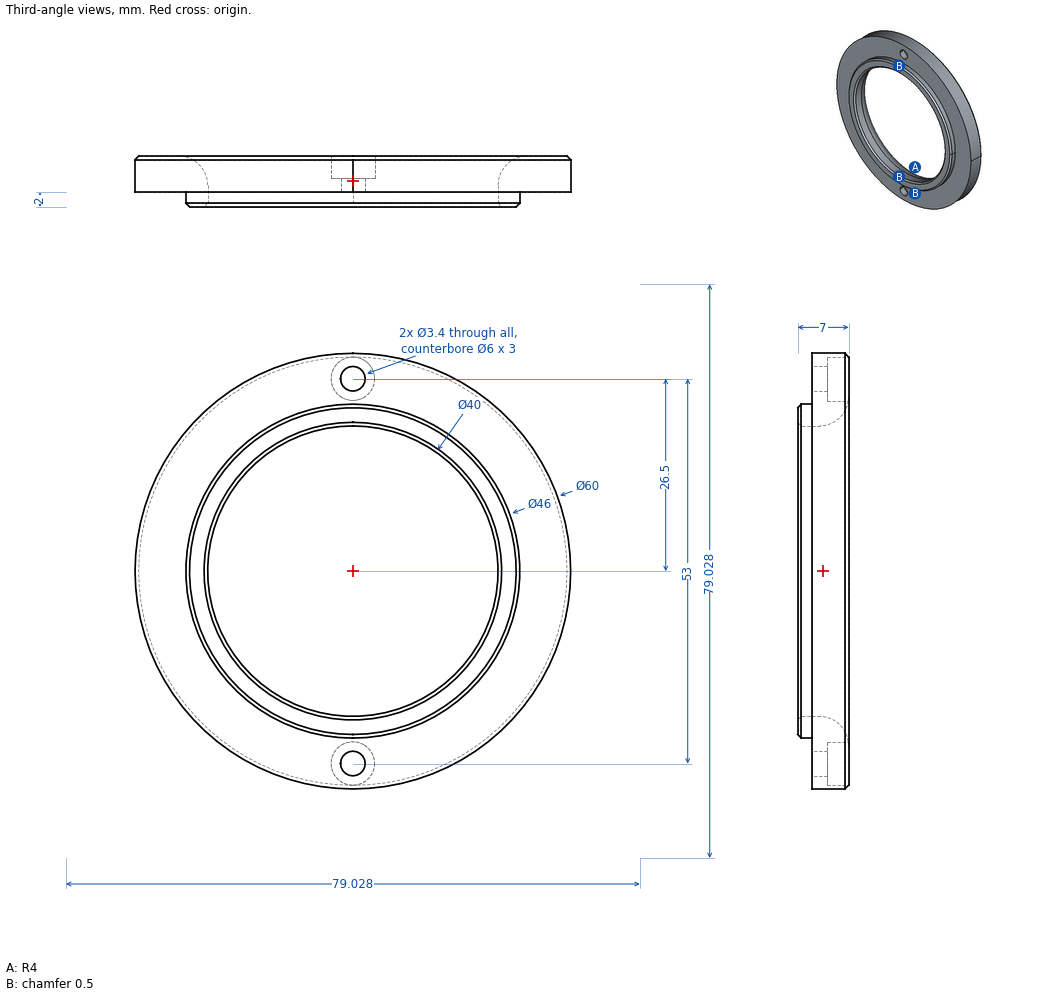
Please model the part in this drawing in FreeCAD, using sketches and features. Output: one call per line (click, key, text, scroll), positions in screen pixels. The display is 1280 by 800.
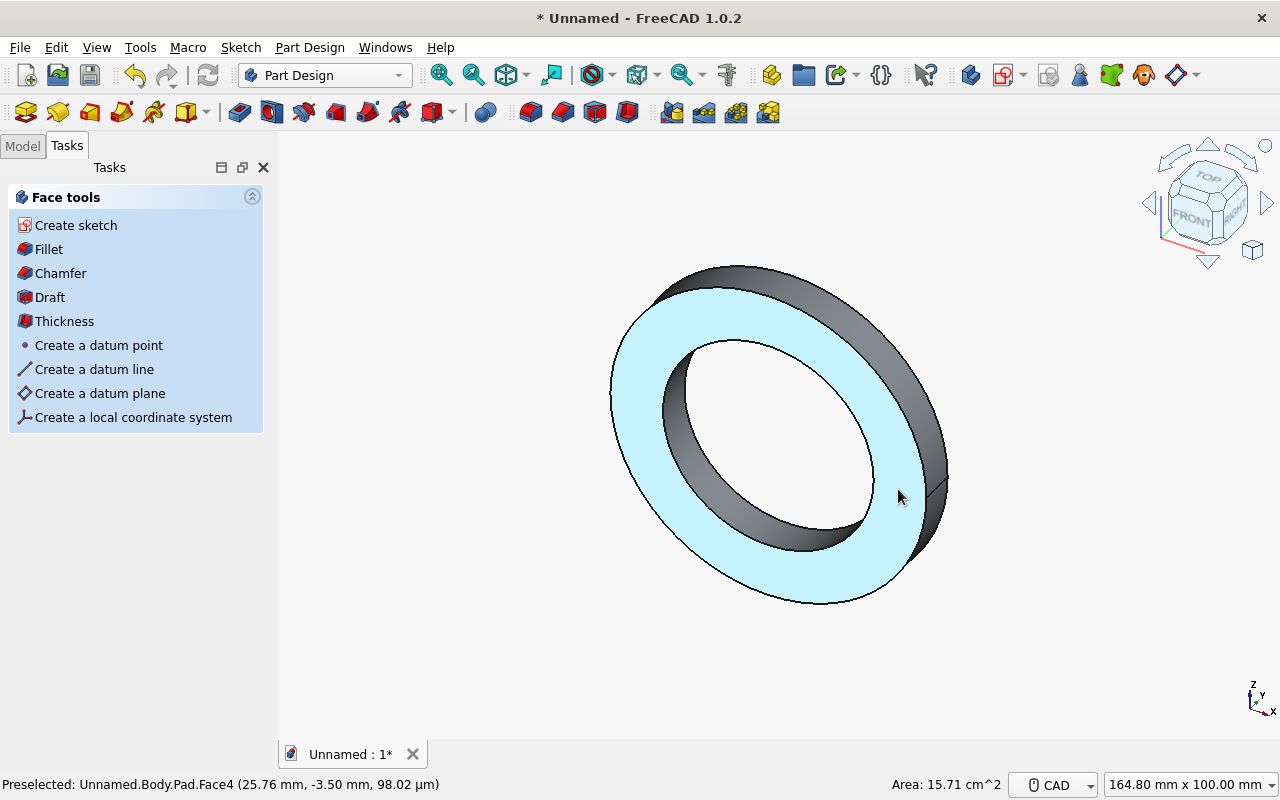
click(1004, 76)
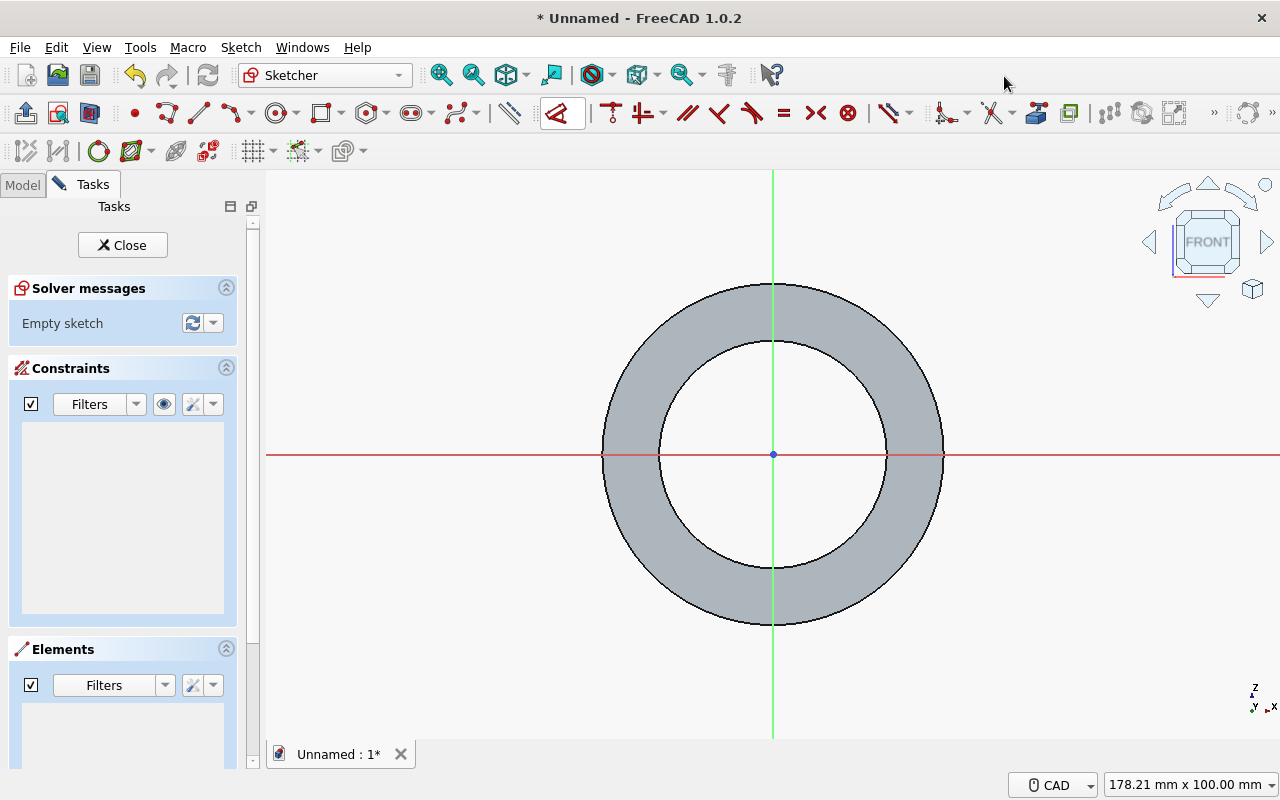
click(344, 114)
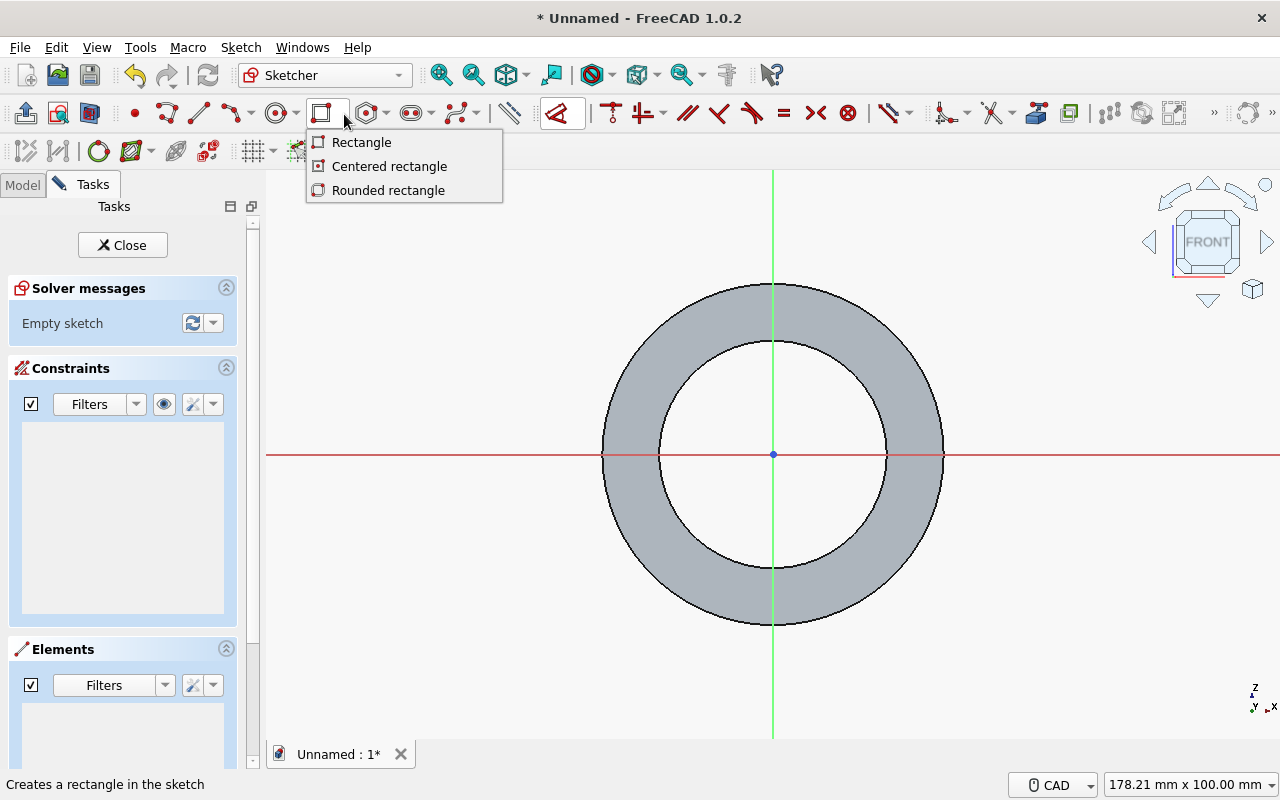
click(404, 166)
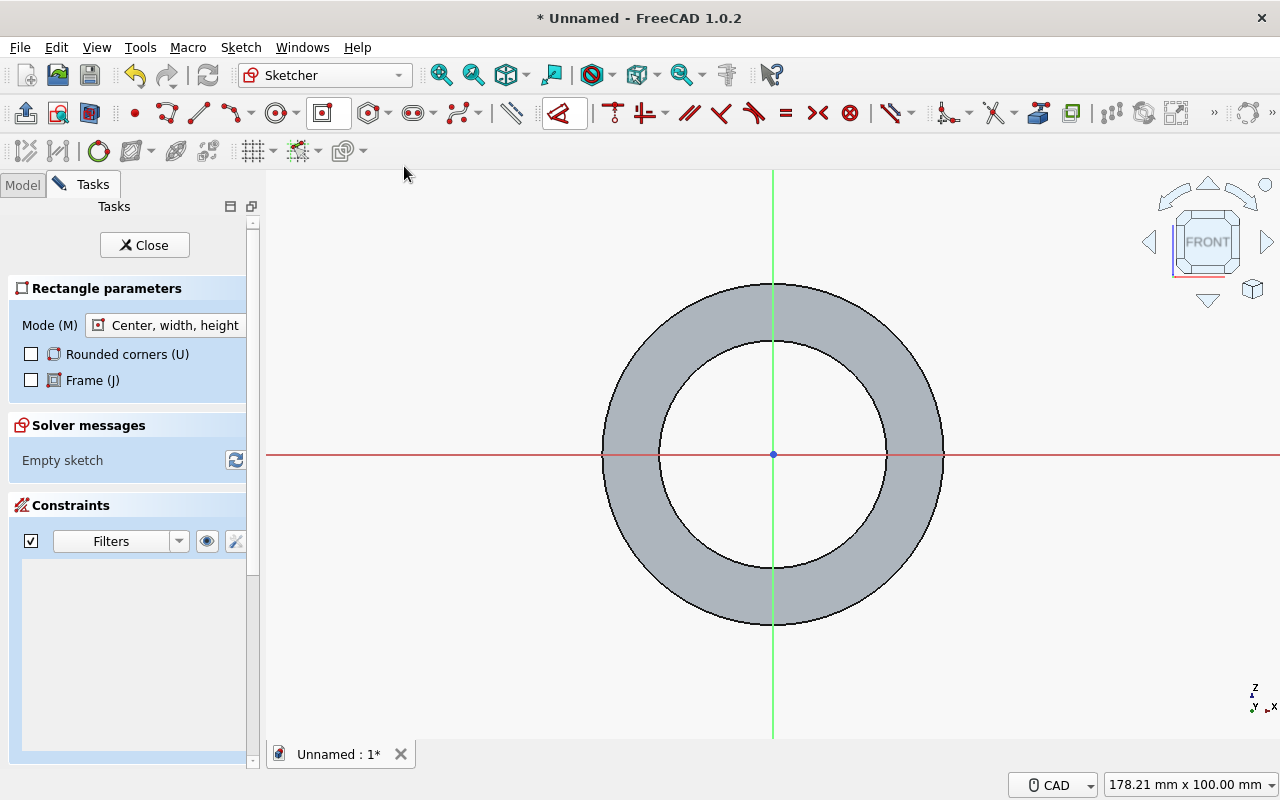
click(773, 454)
click(998, 230)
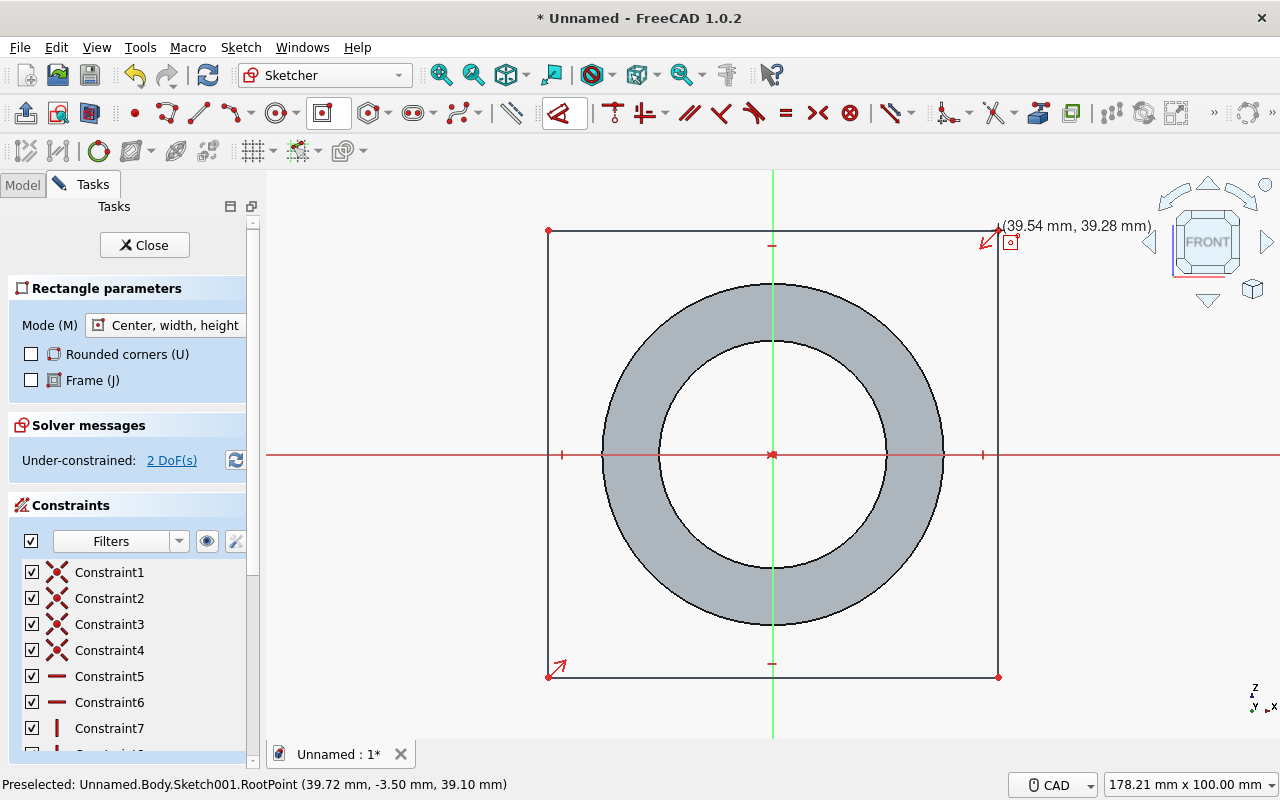
click(276, 114)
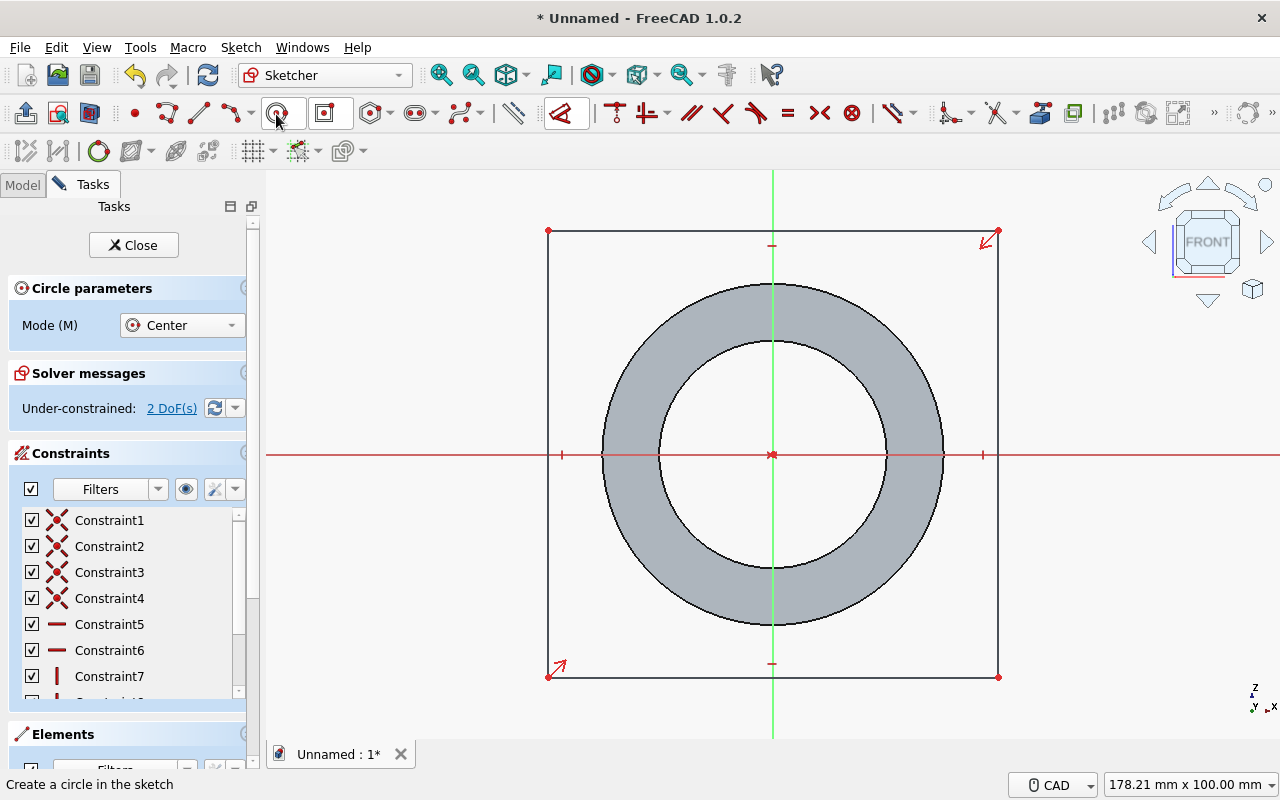
click(773, 454)
click(866, 362)
key(Escape)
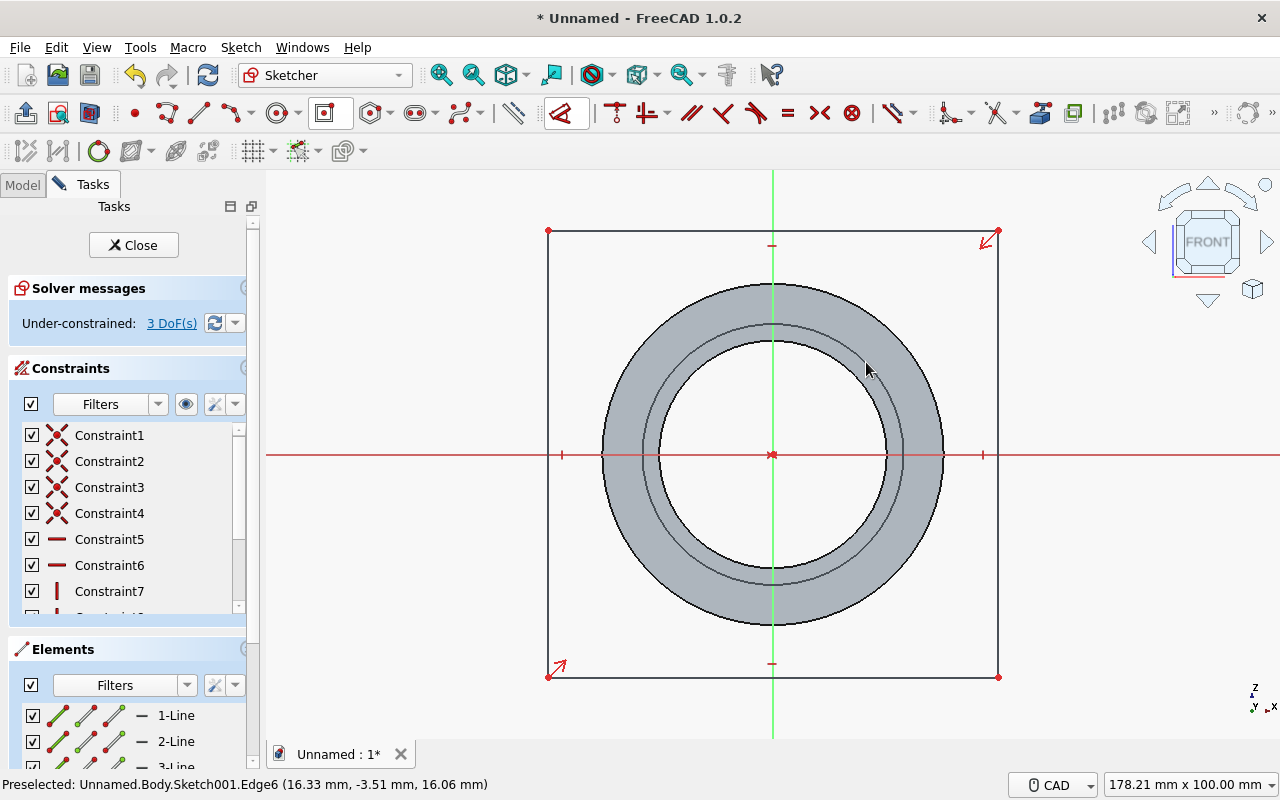
click(865, 362)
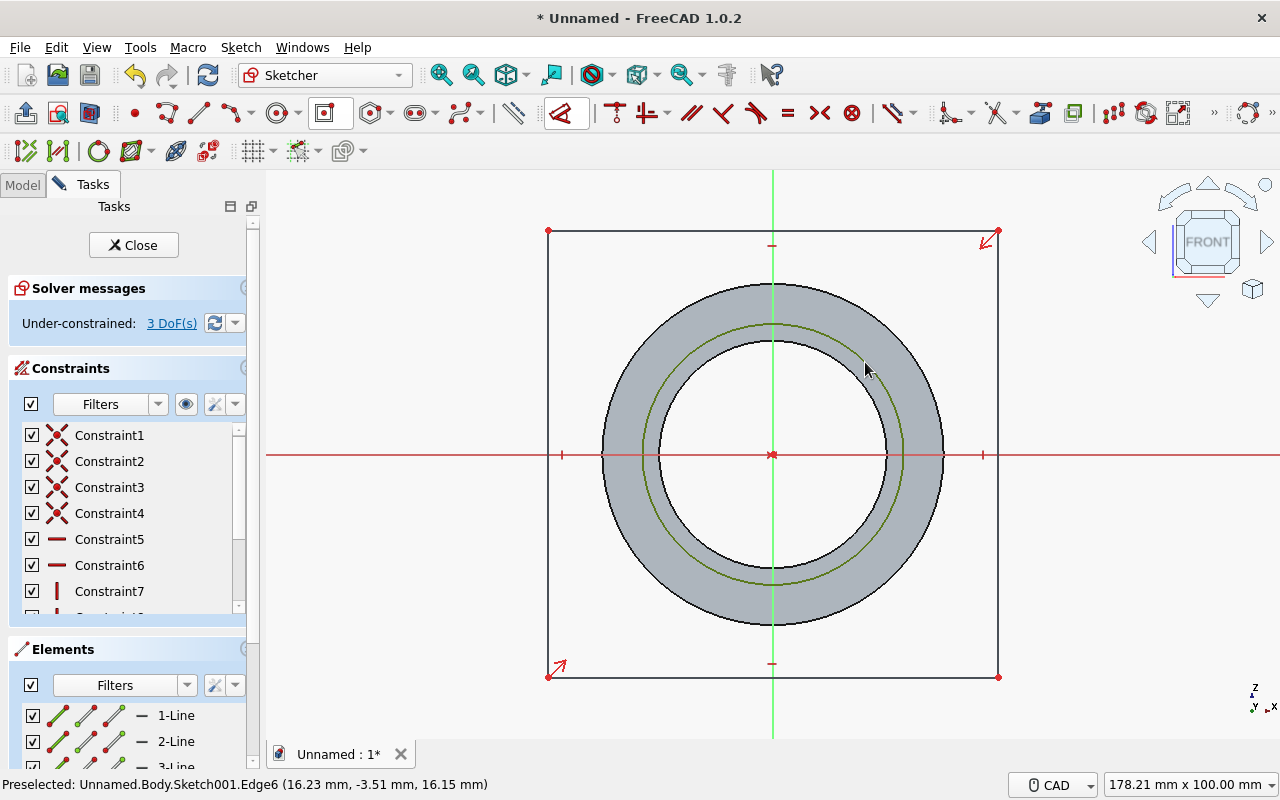
key(k)
key(o)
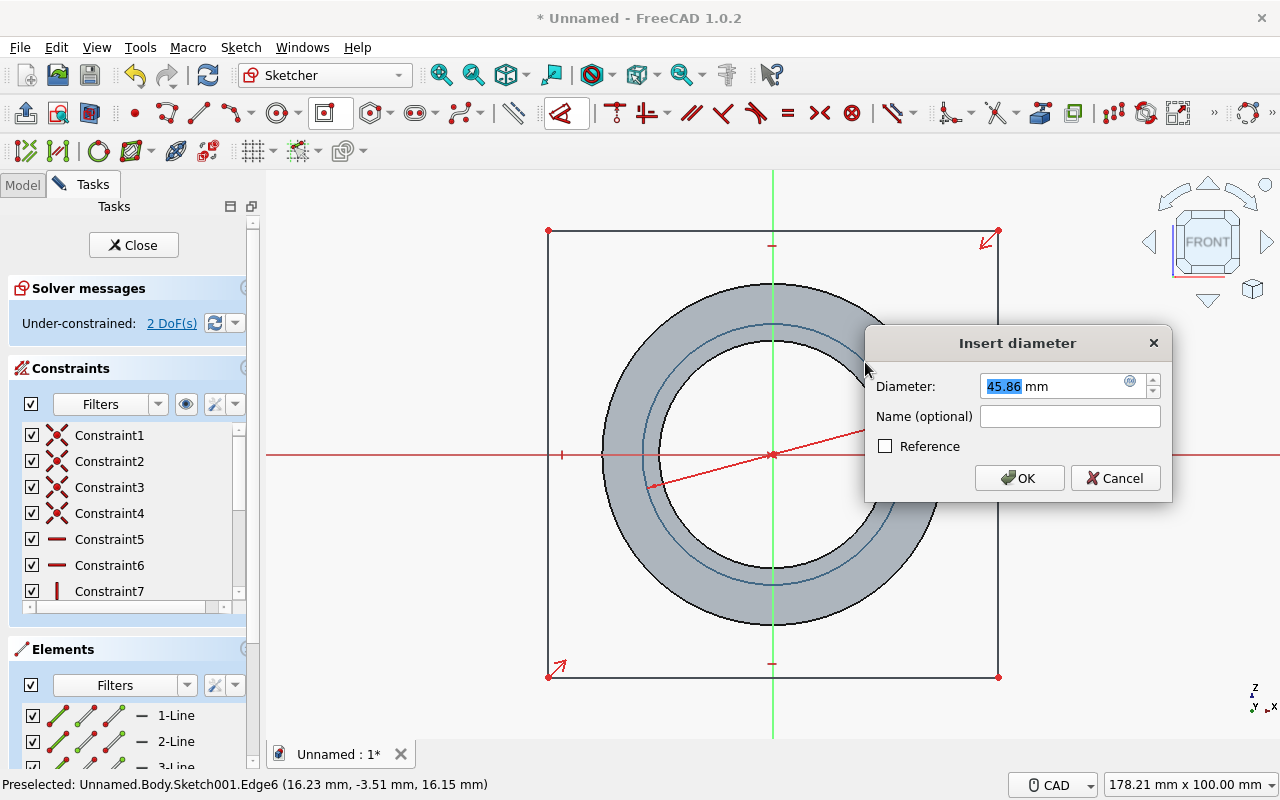
text(46)
key(Return)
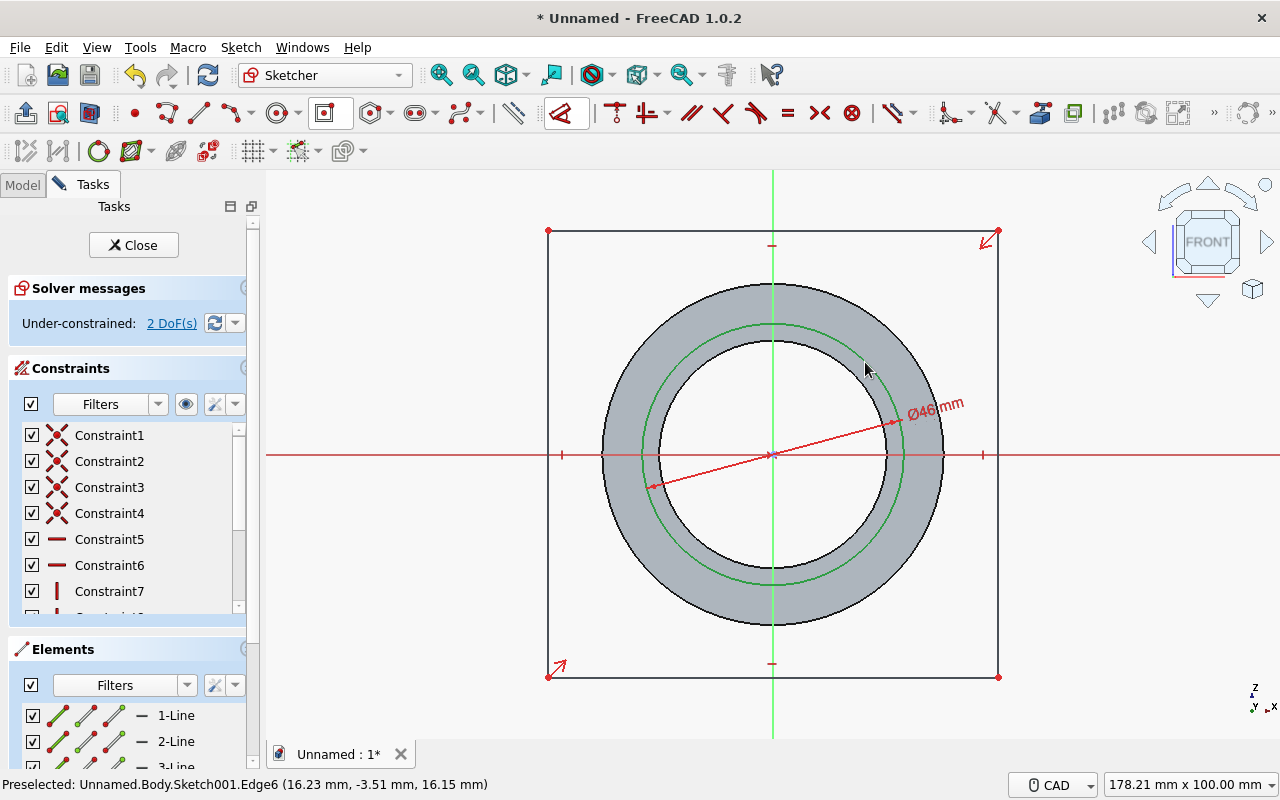
click(683, 678)